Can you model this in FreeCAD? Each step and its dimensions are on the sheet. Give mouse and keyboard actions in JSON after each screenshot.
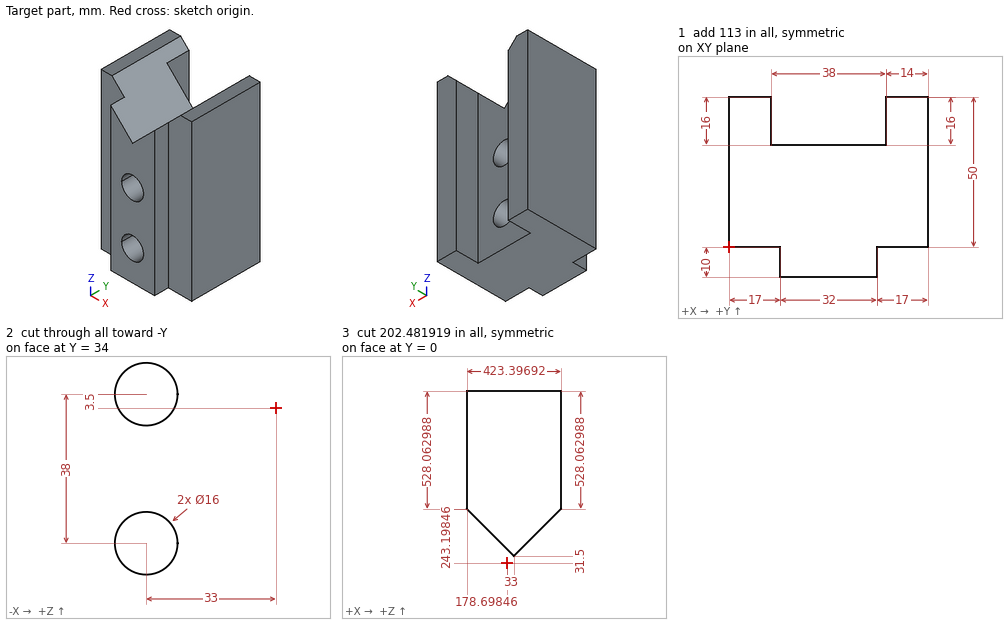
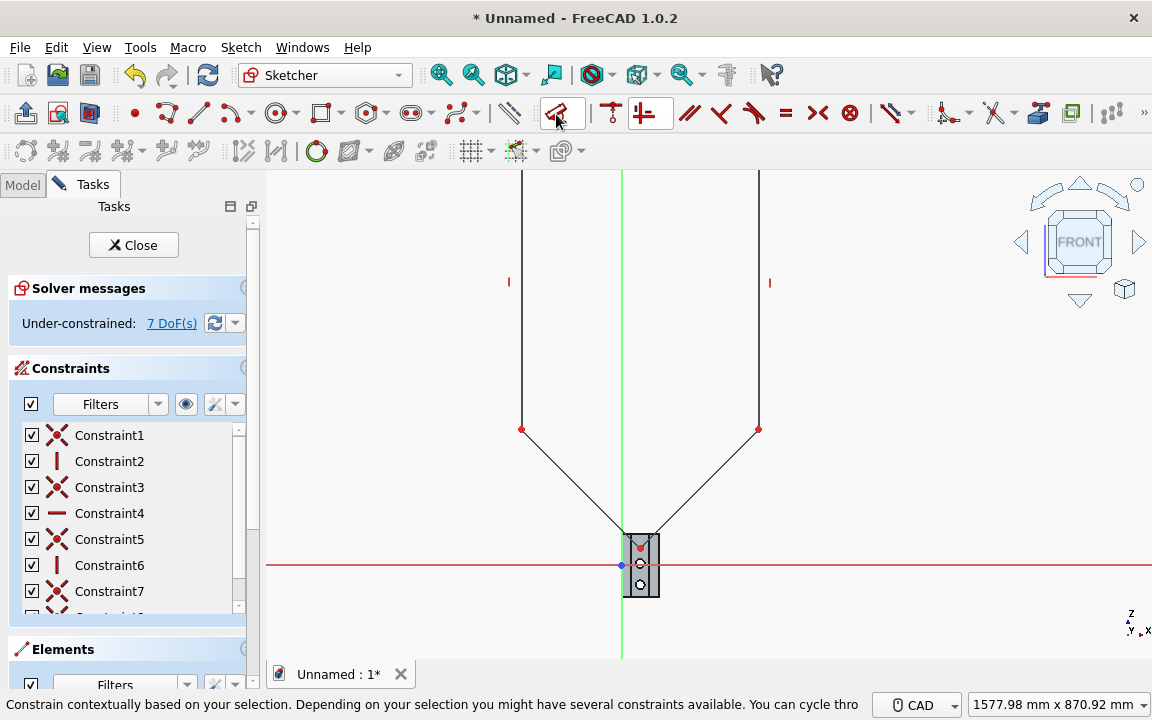
{"action": "scroll", "coordinate": [641, 549], "scroll_direction": "up", "scroll_amount": 4}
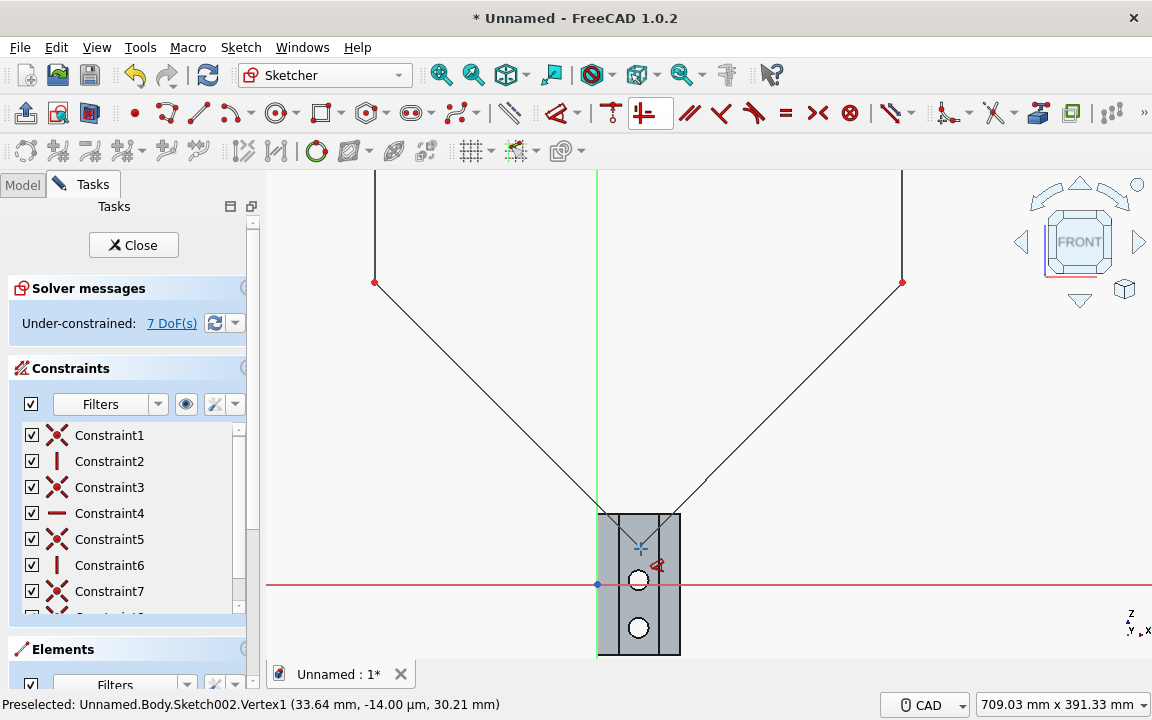
{"action": "left_click", "coordinate": [639, 547]}
{"action": "left_click", "coordinate": [618, 619]}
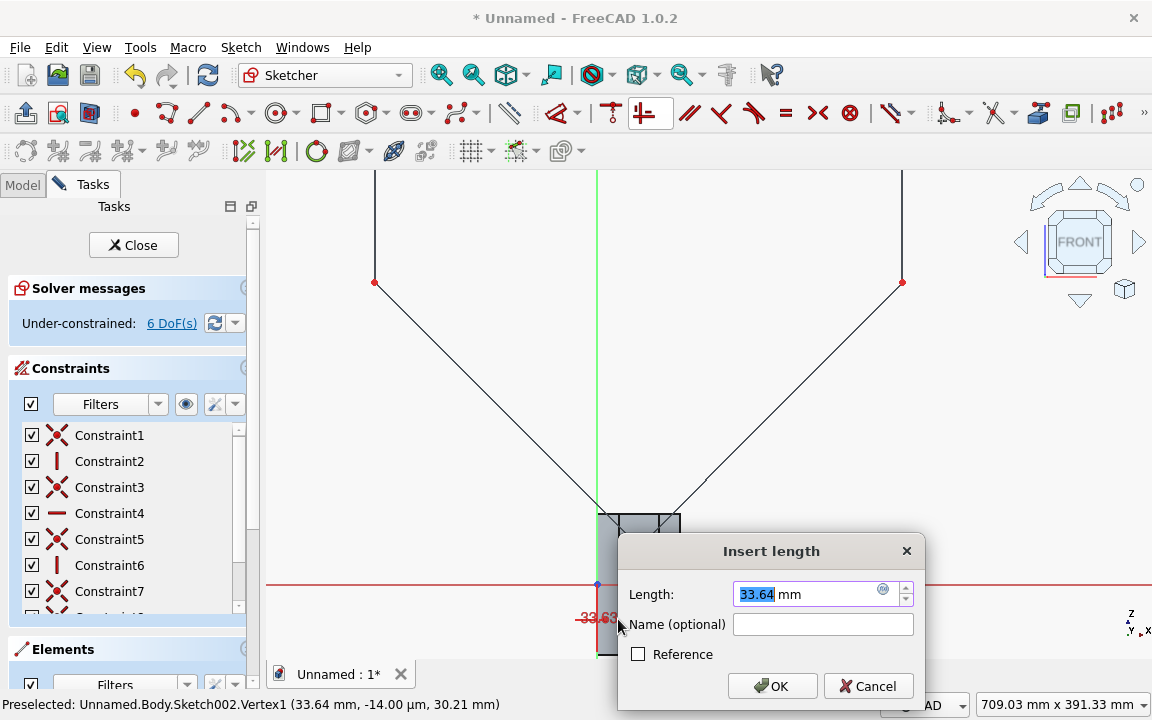
{"action": "type", "text": "33"}
{"action": "key", "text": "Return"}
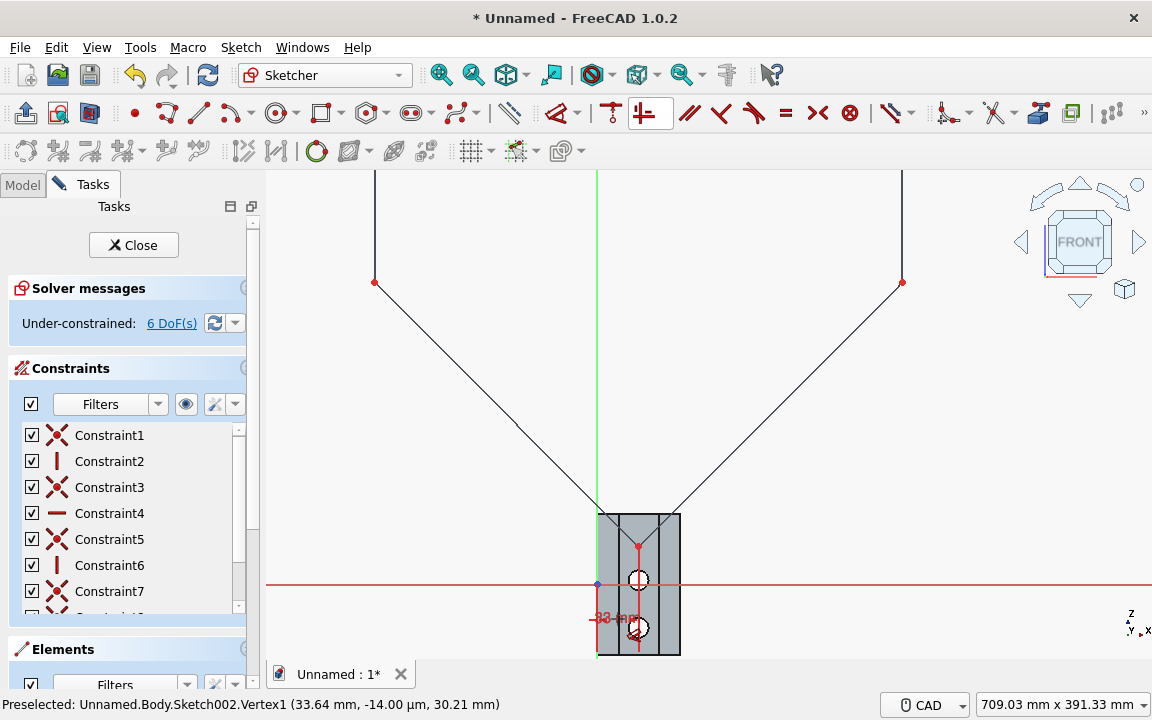
{"action": "left_click", "coordinate": [639, 547]}
{"action": "left_click", "coordinate": [563, 566]}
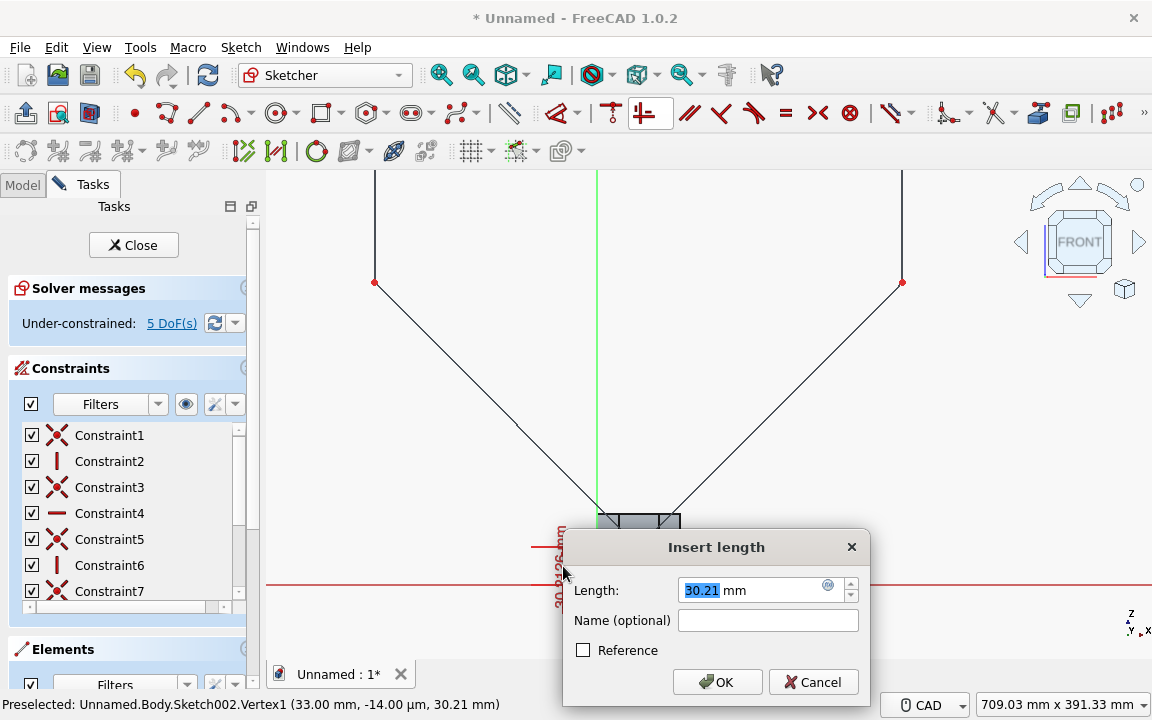
{"action": "type", "text": "31.5"}
{"action": "key", "text": "Return"}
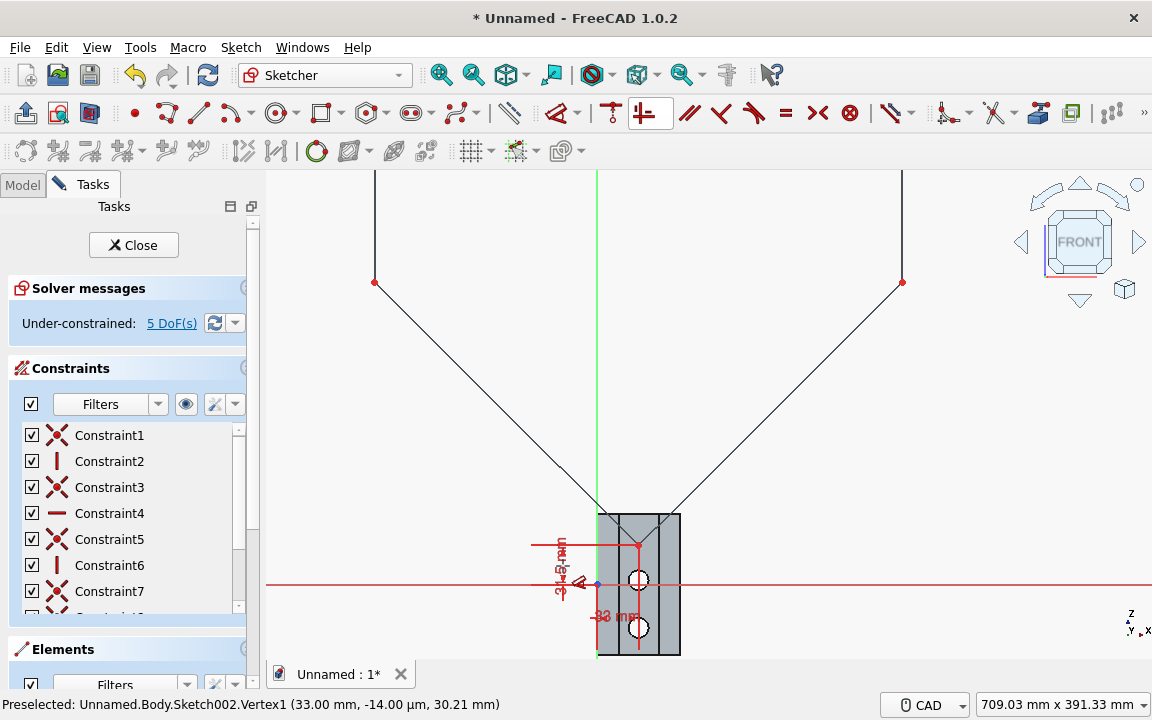
{"action": "scroll", "coordinate": [641, 549], "scroll_direction": "down", "scroll_amount": 6}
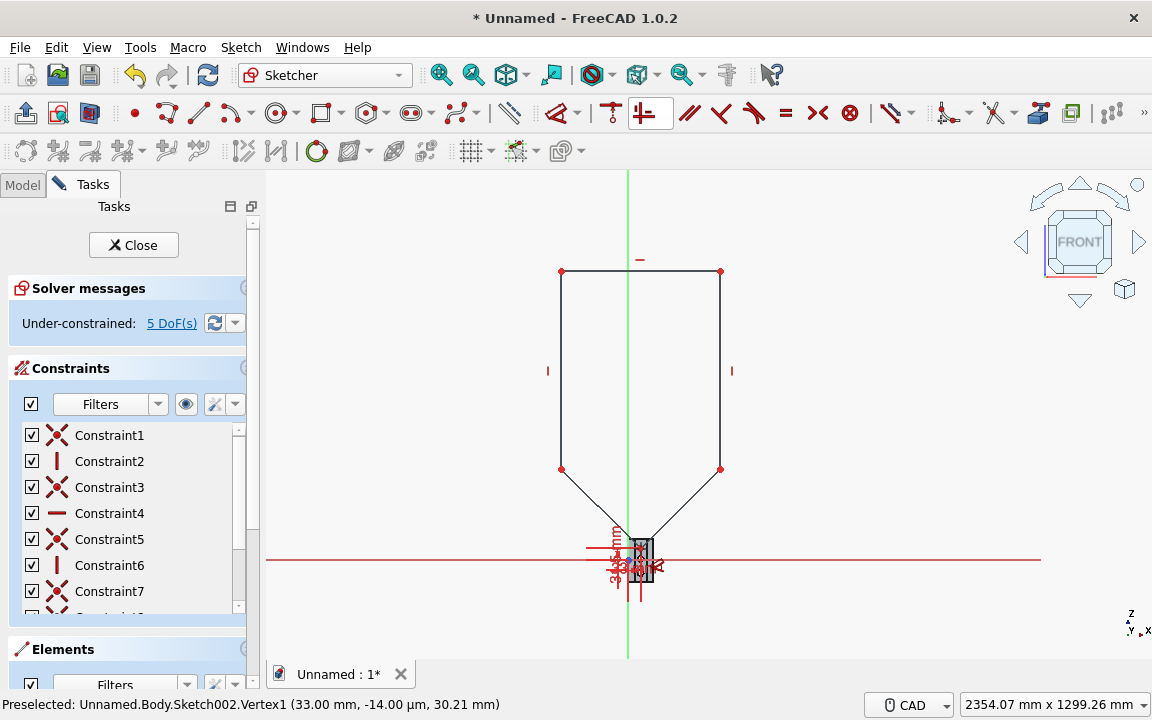
{"action": "left_click", "coordinate": [609, 271]}
{"action": "left_click", "coordinate": [604, 237]}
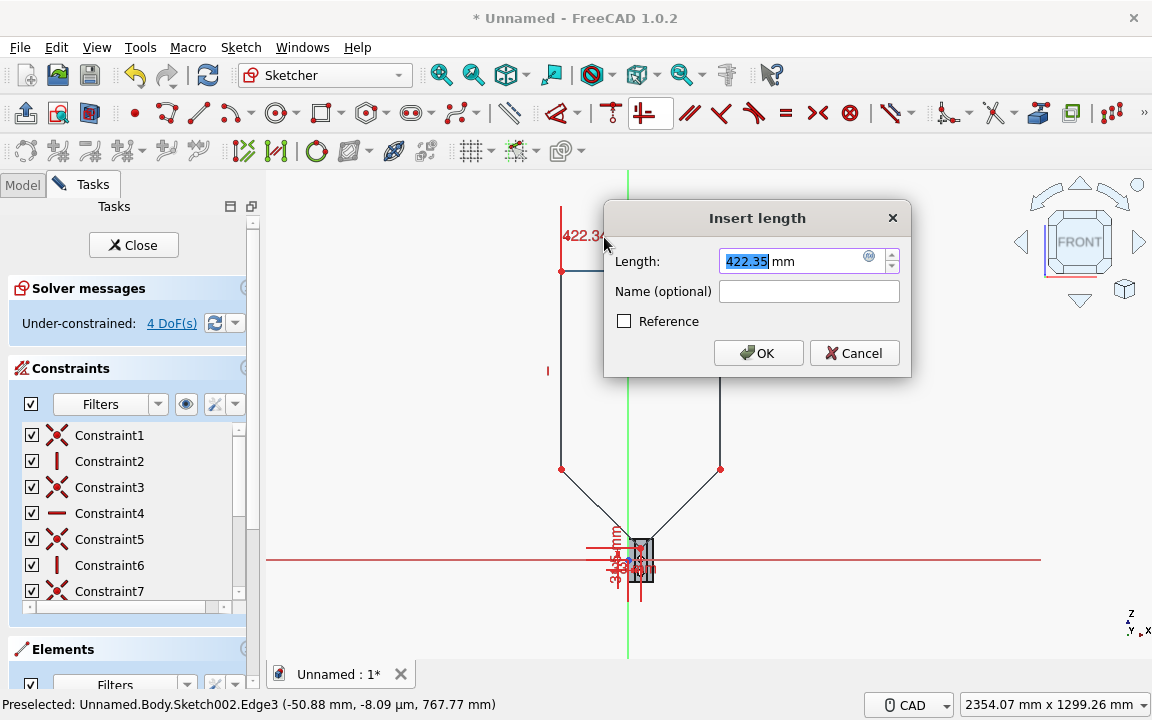
{"action": "type", "text": "423.39692"}
{"action": "key", "text": "Return"}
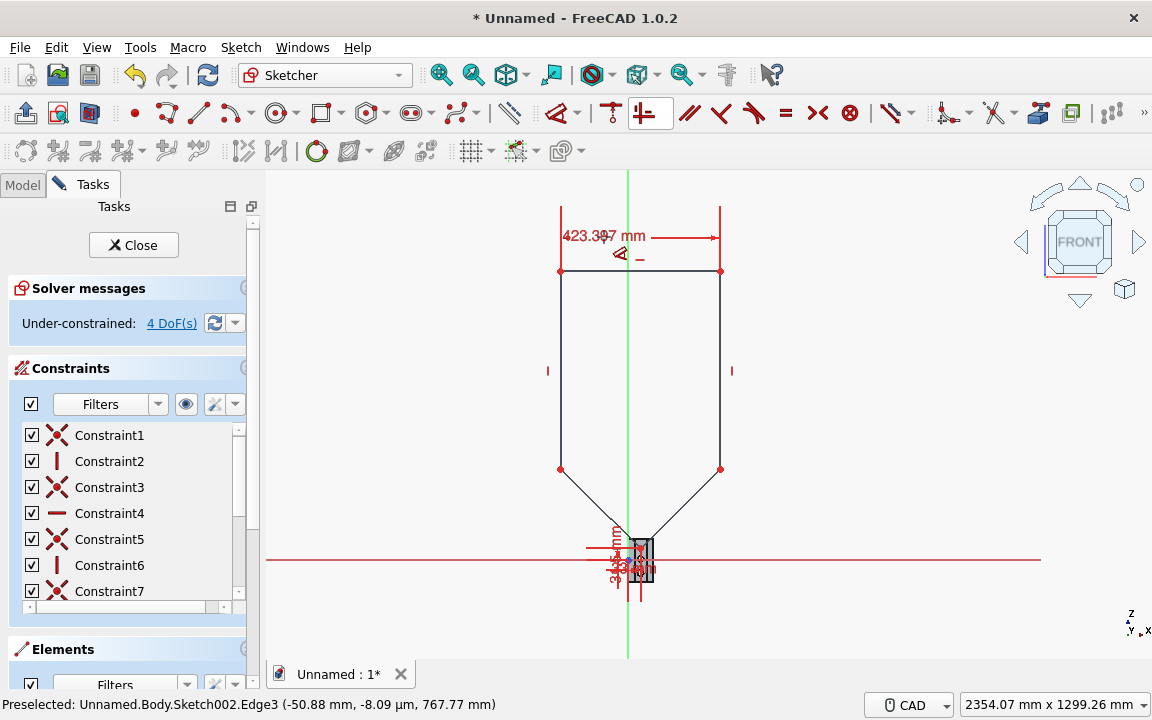
{"action": "left_click", "coordinate": [561, 410]}
{"action": "left_click", "coordinate": [527, 370]}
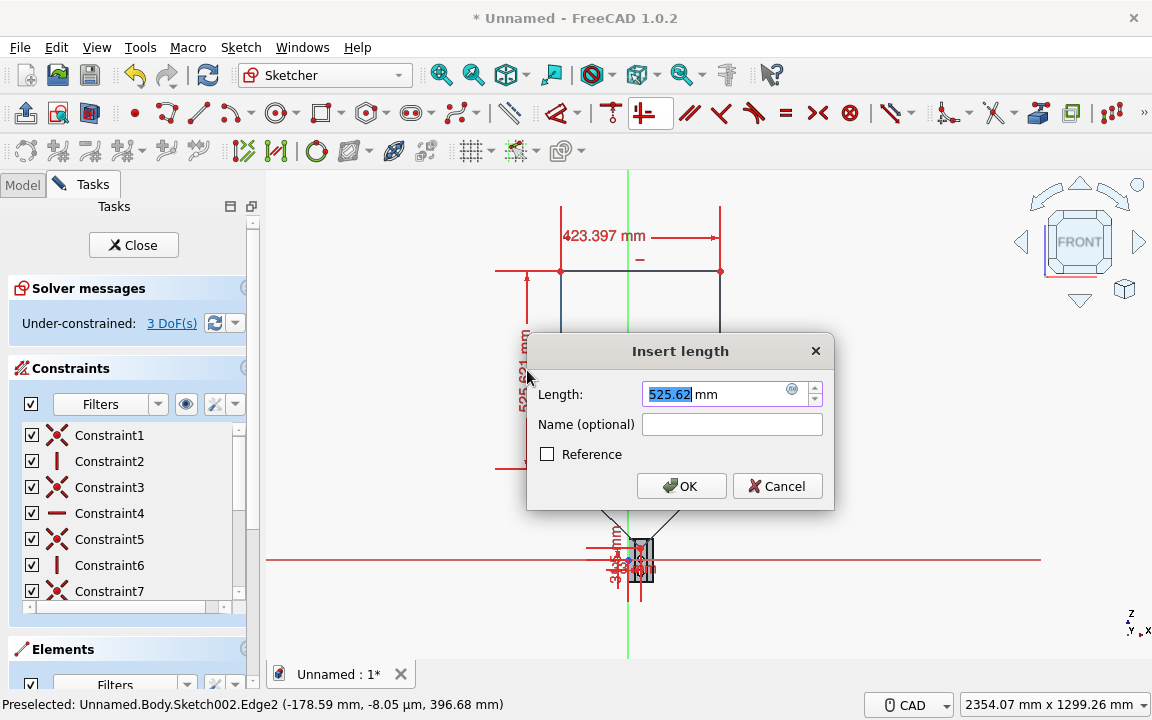
{"action": "type", "text": "528.062988"}
{"action": "key", "text": "Return"}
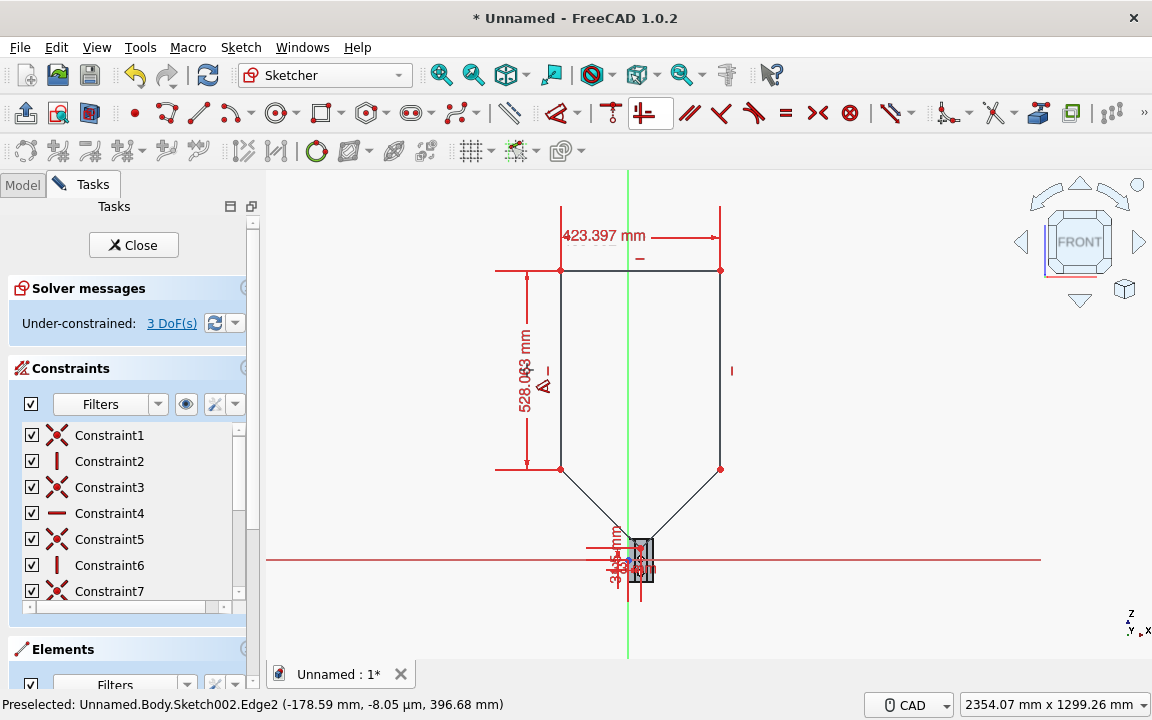
{"action": "left_click", "coordinate": [720, 330]}
{"action": "left_click", "coordinate": [754, 370]}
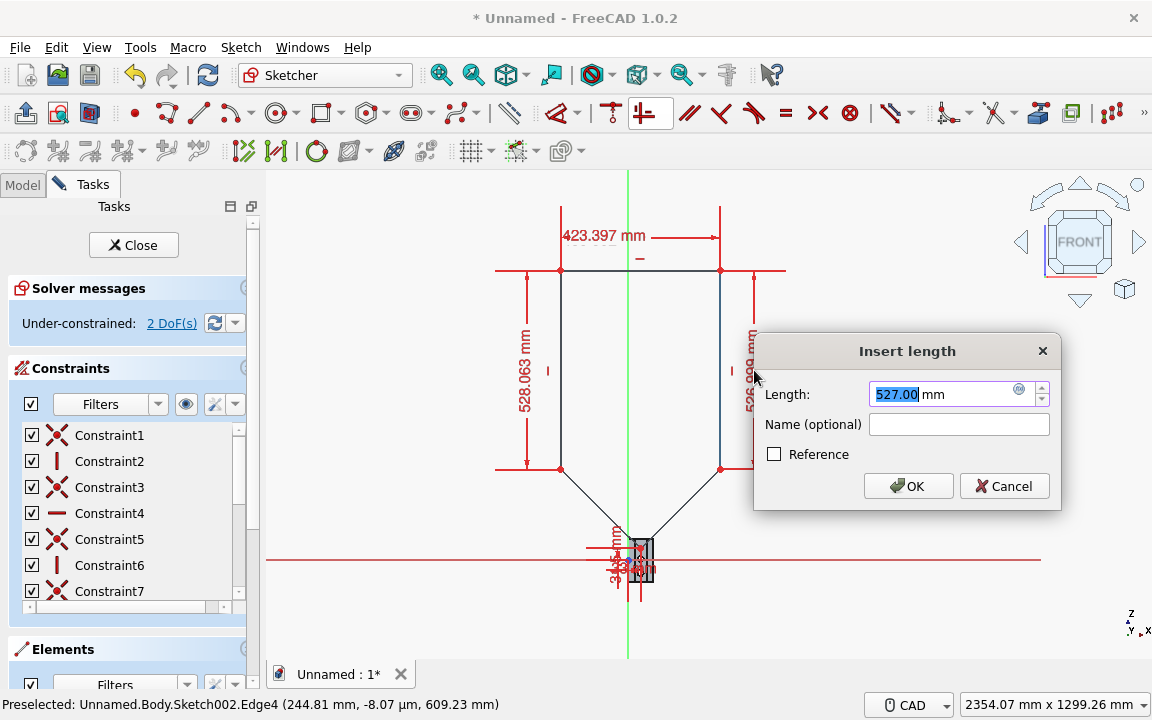
{"action": "type", "text": "528.062988"}
{"action": "key", "text": "Return"}